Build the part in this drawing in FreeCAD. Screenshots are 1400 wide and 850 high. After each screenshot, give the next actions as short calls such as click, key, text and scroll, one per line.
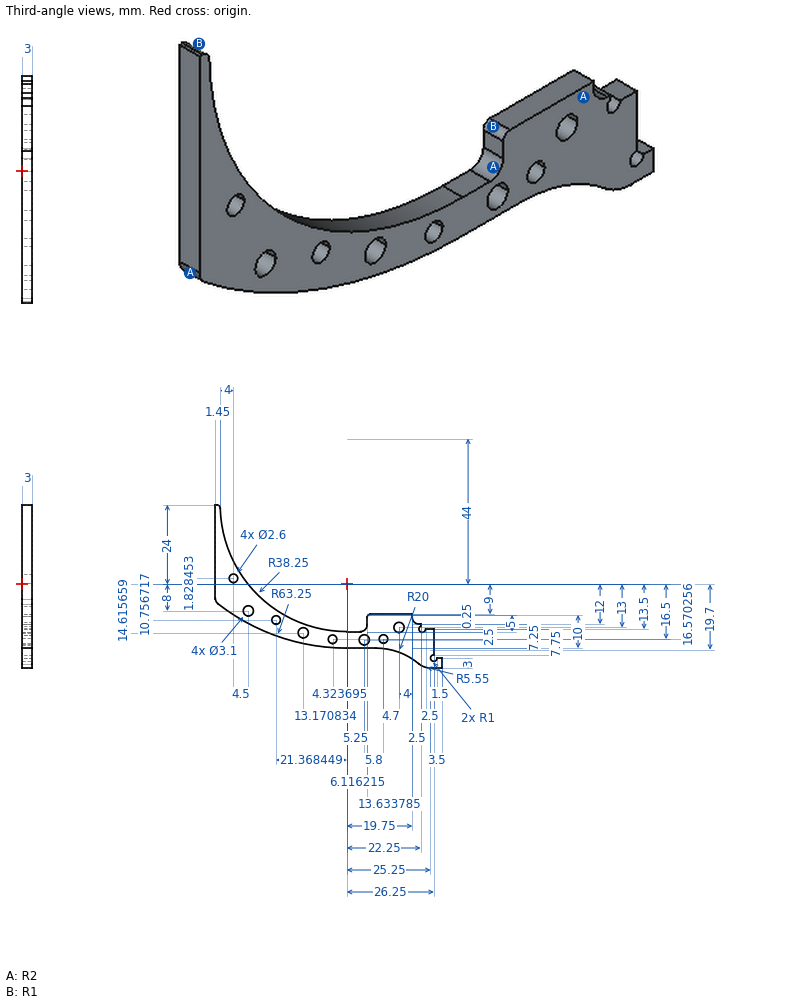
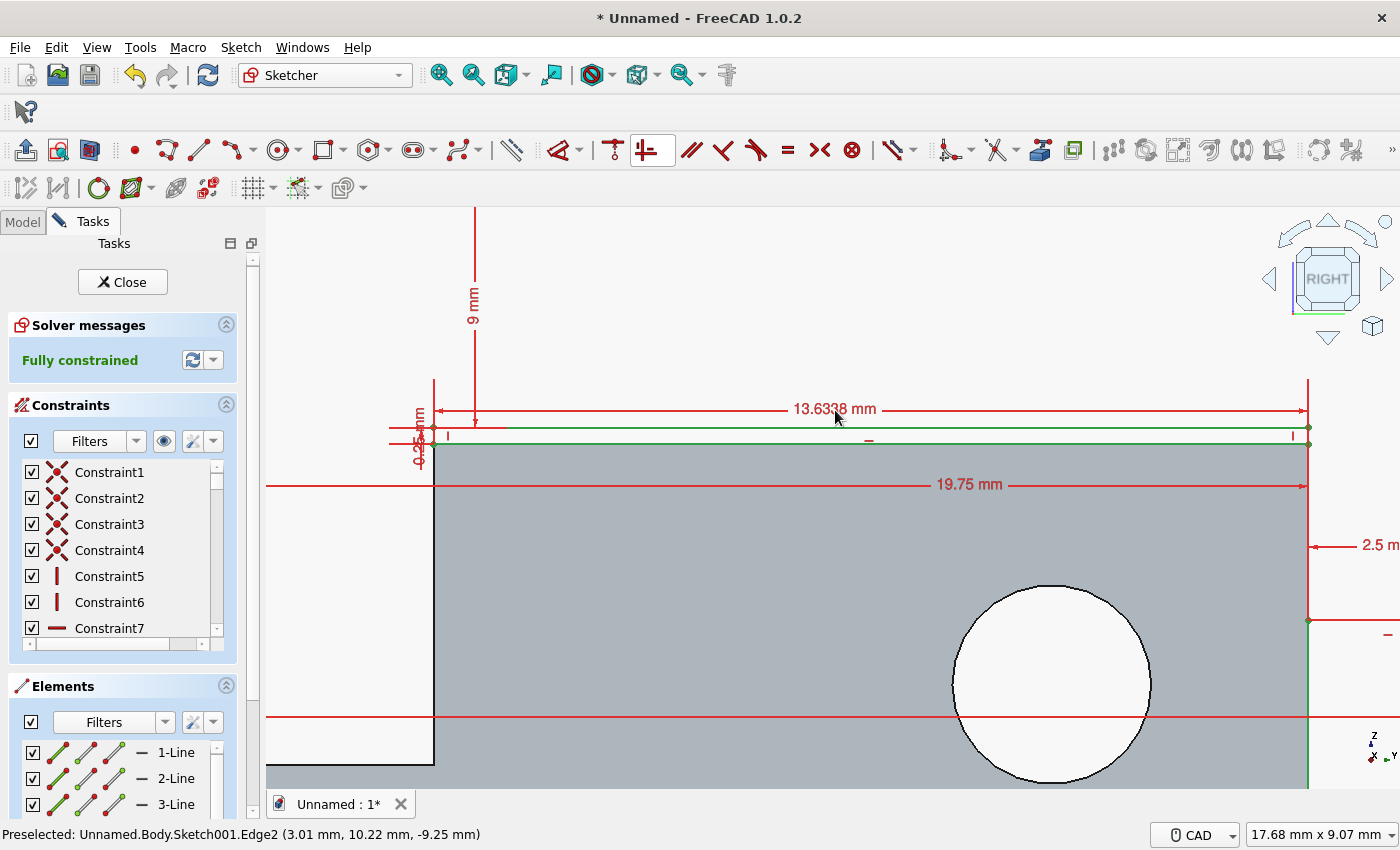
click(123, 282)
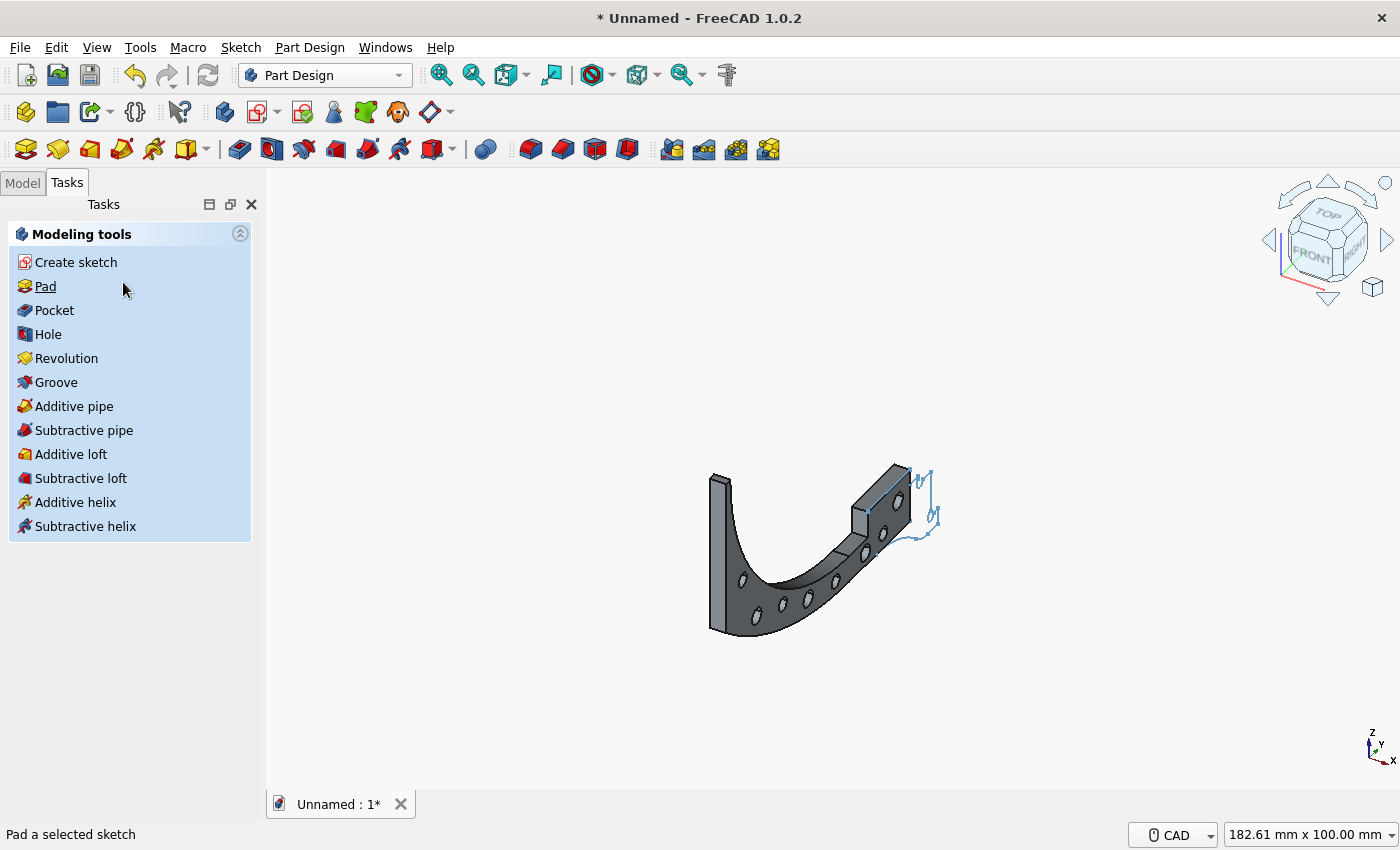
click(26, 150)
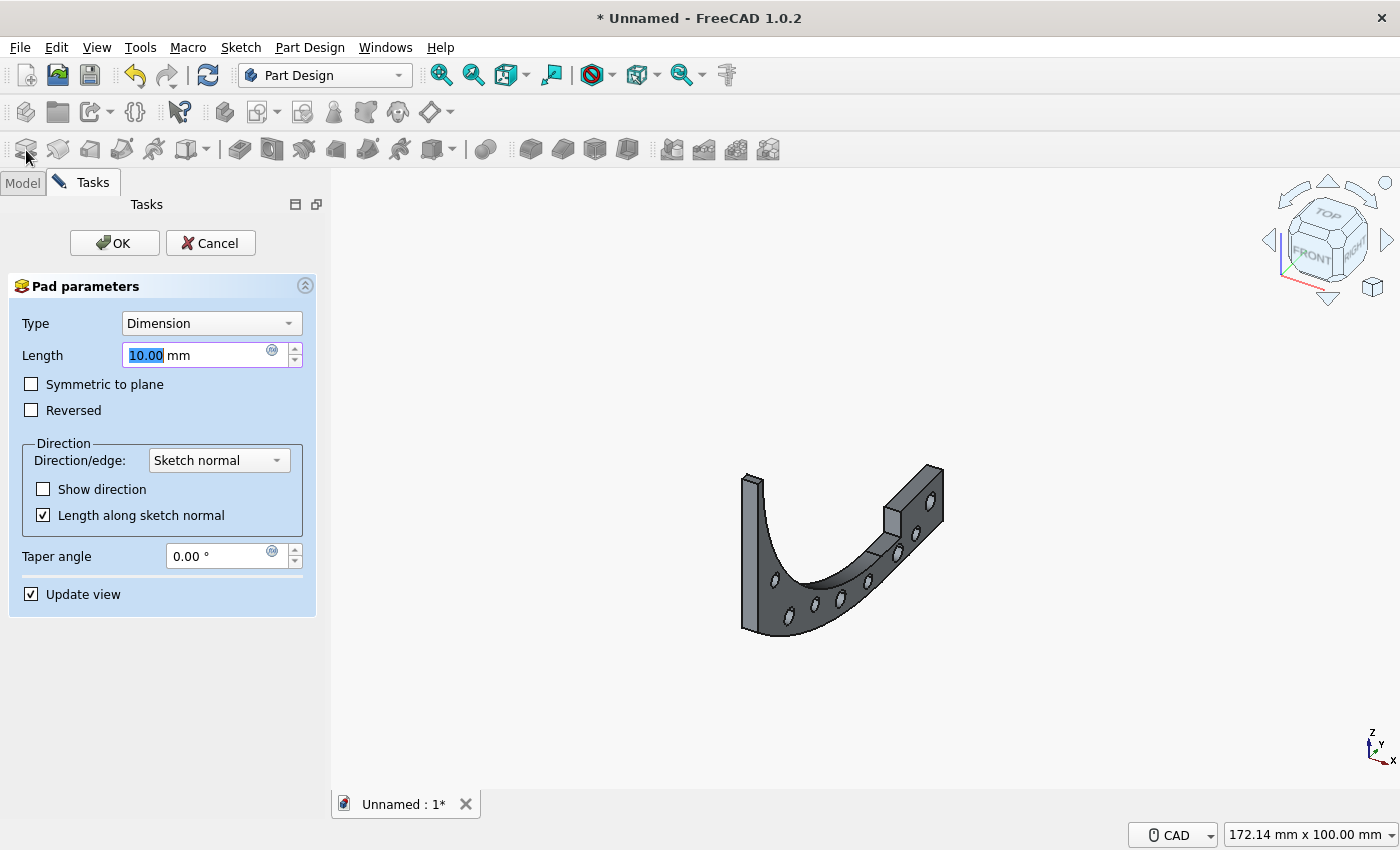
text(3)
key(Tab)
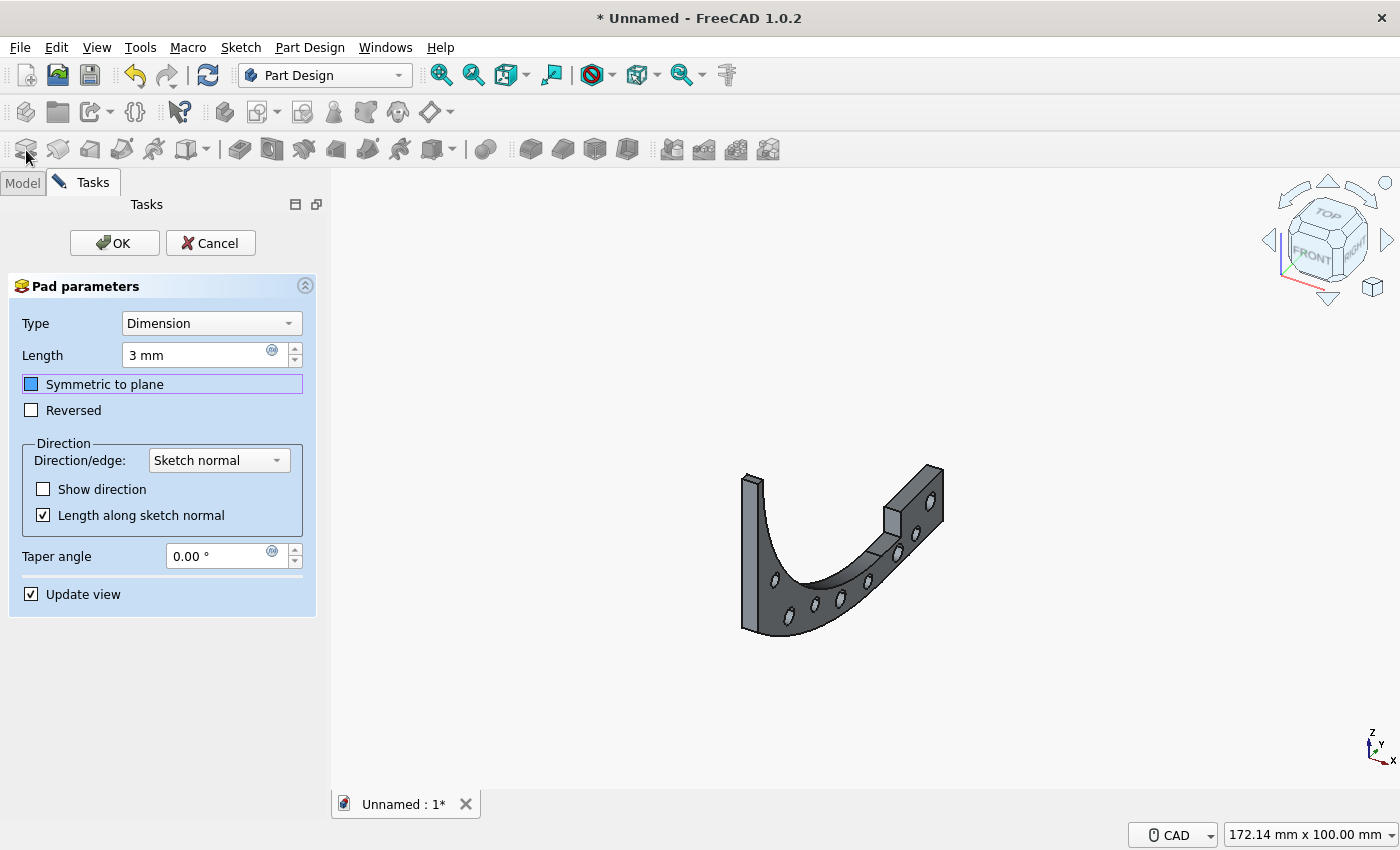
click(30, 410)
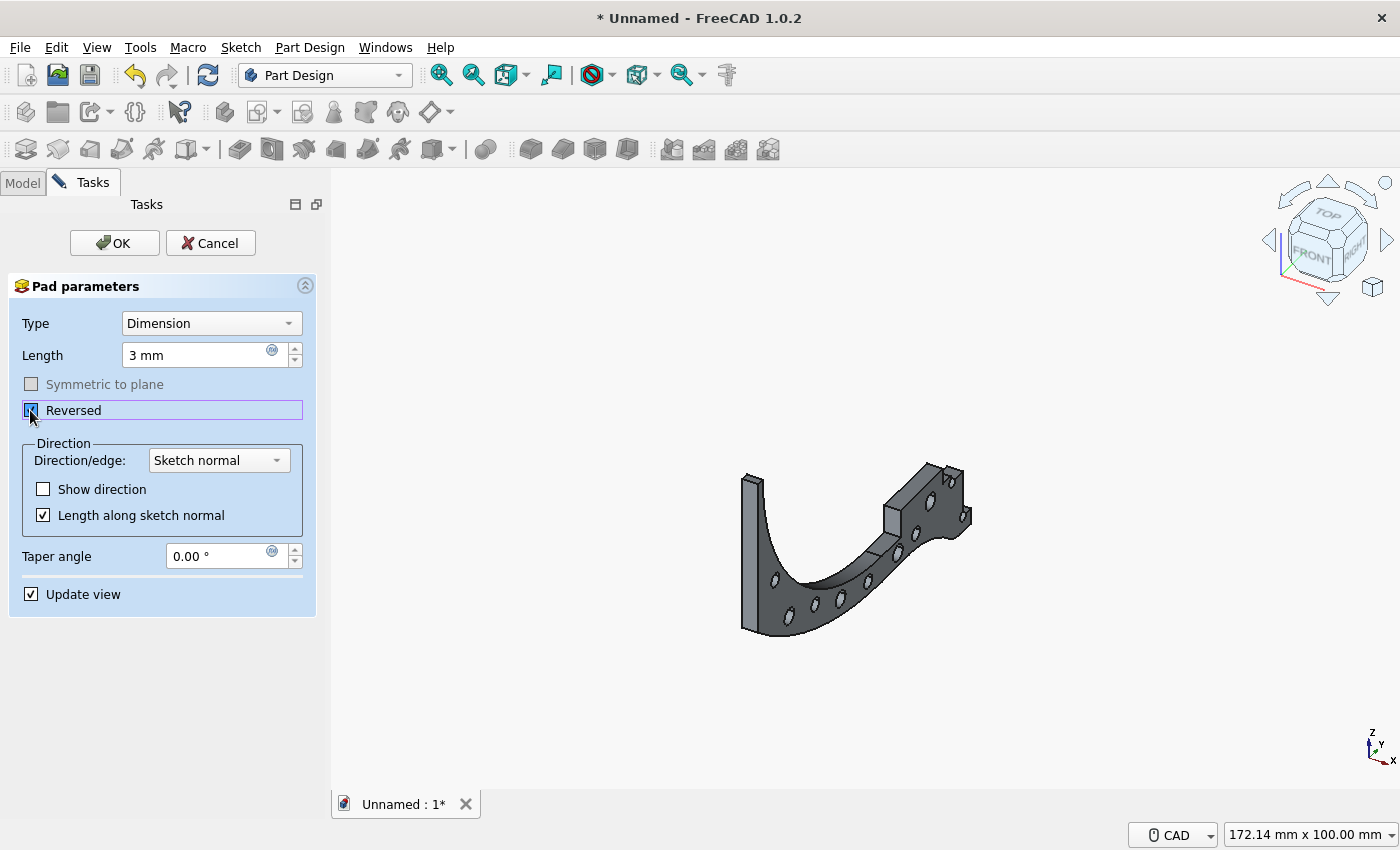
click(115, 243)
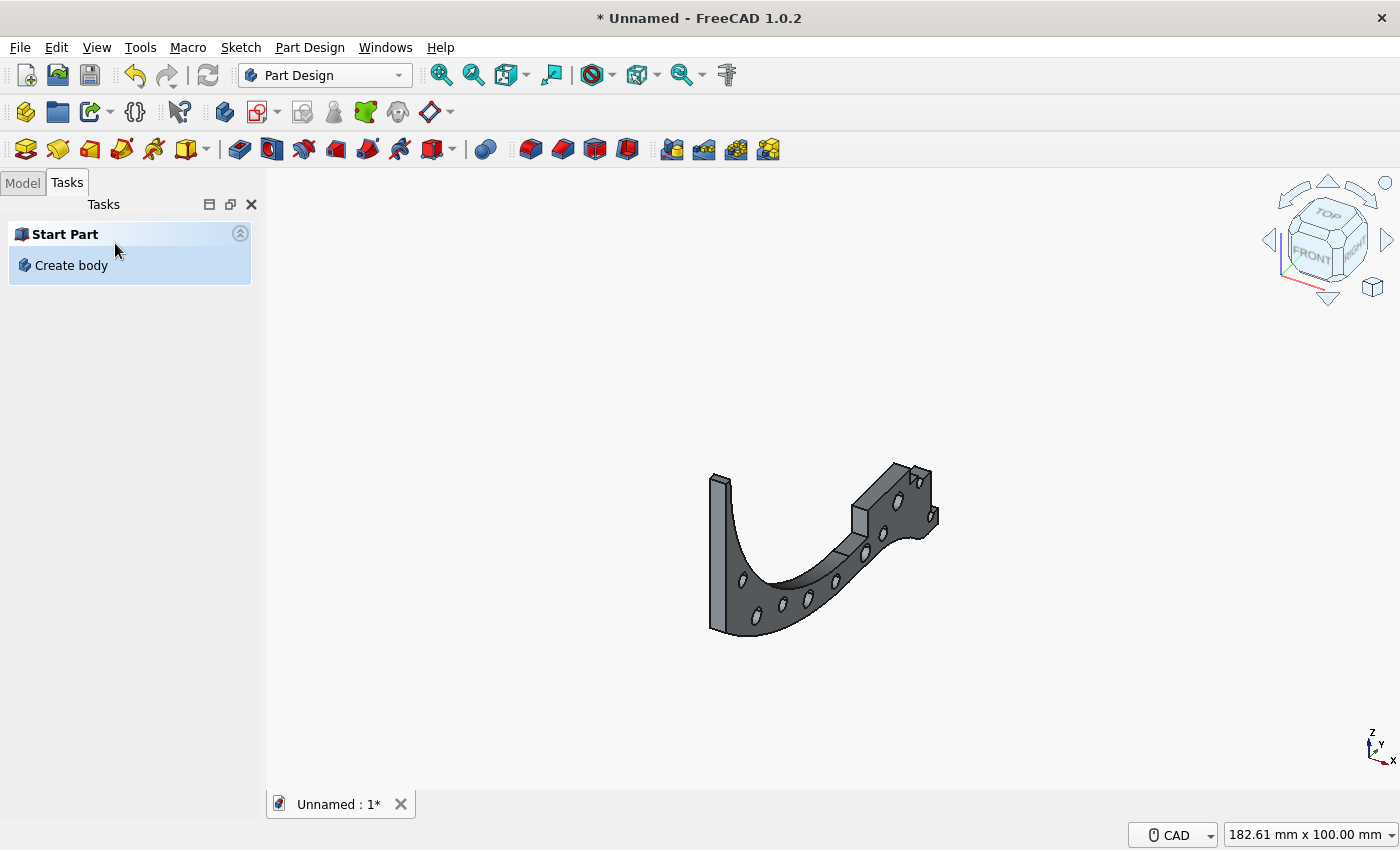
scroll(718, 629, up, 4)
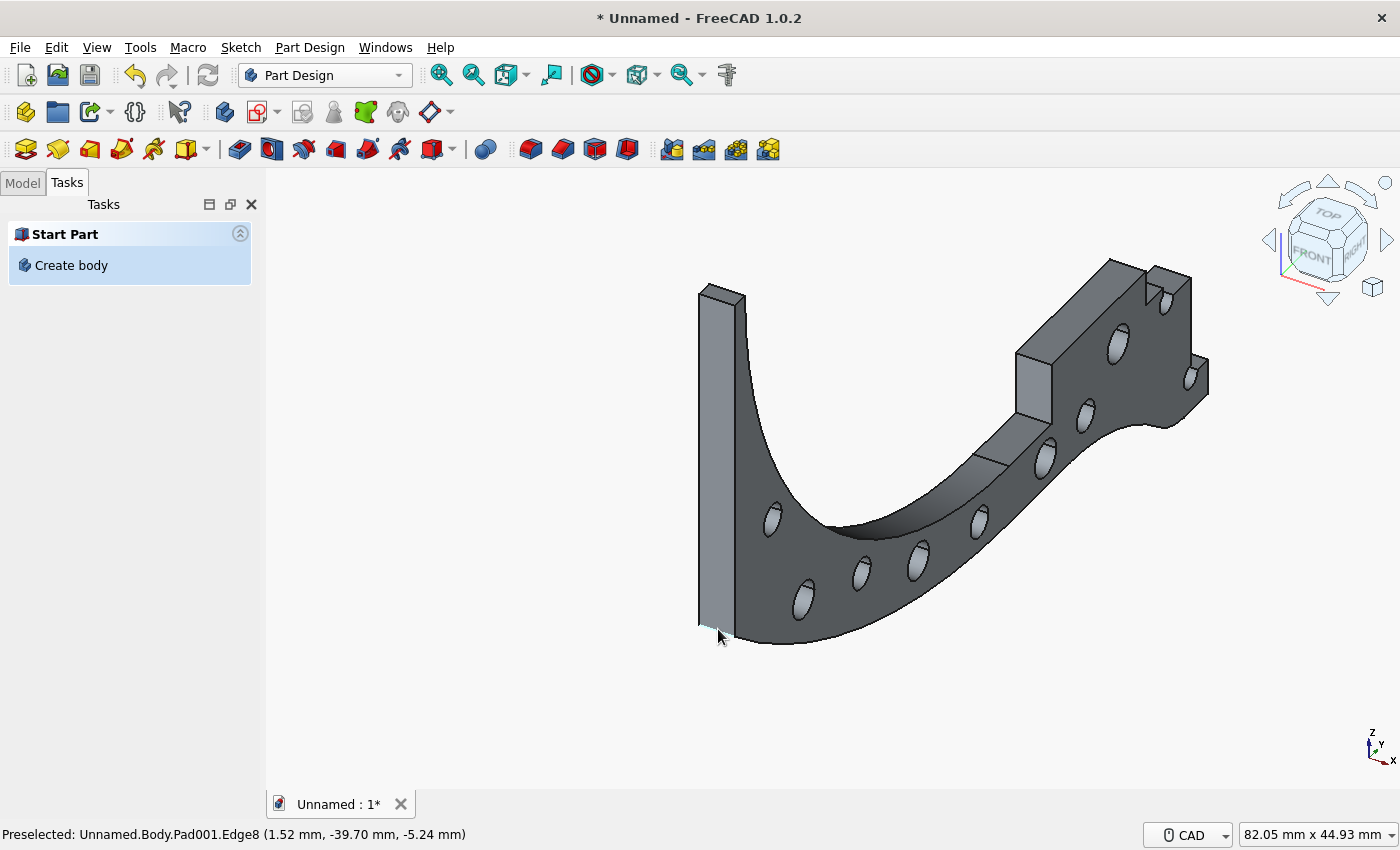
key(v)
key(f)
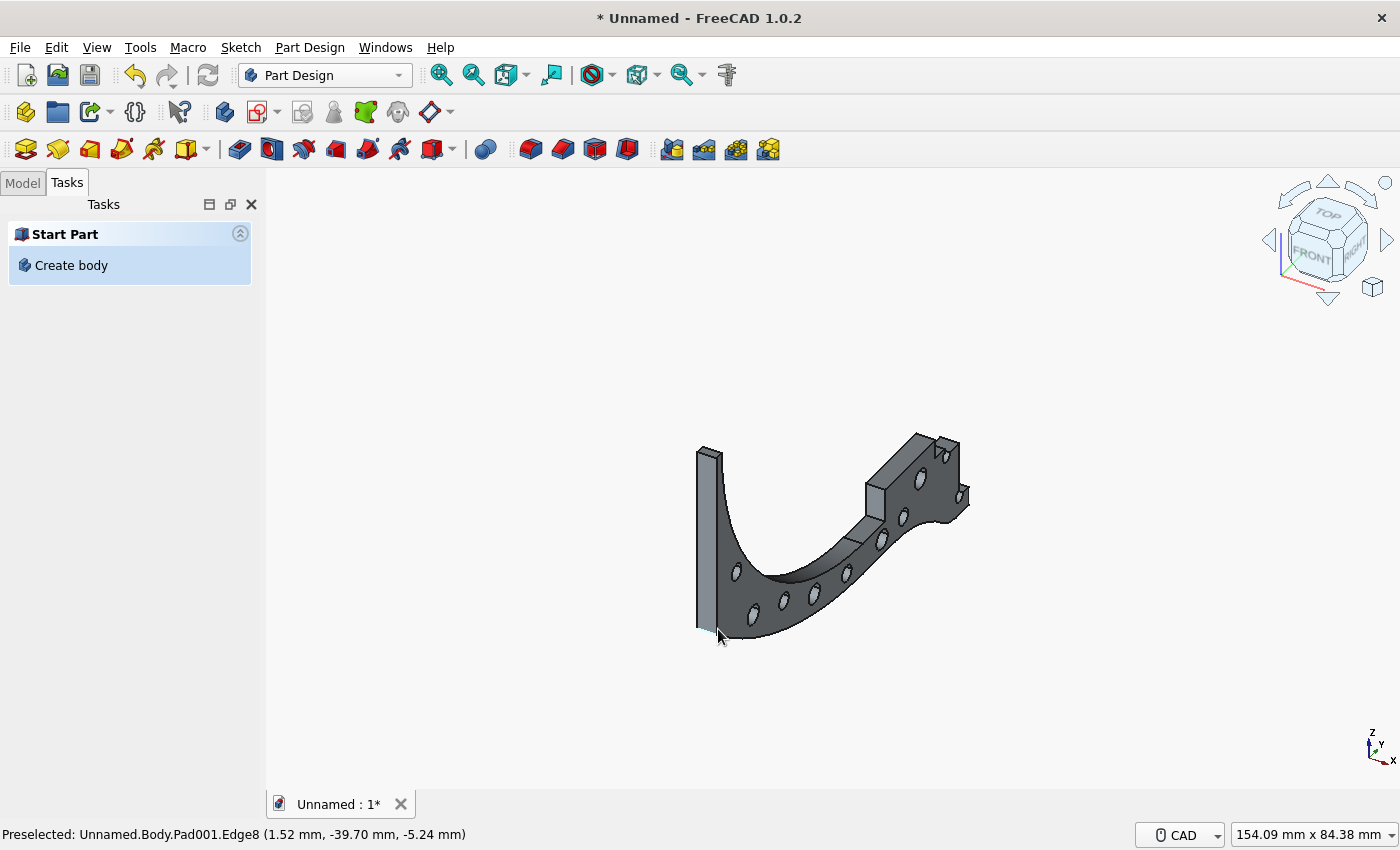
key(0)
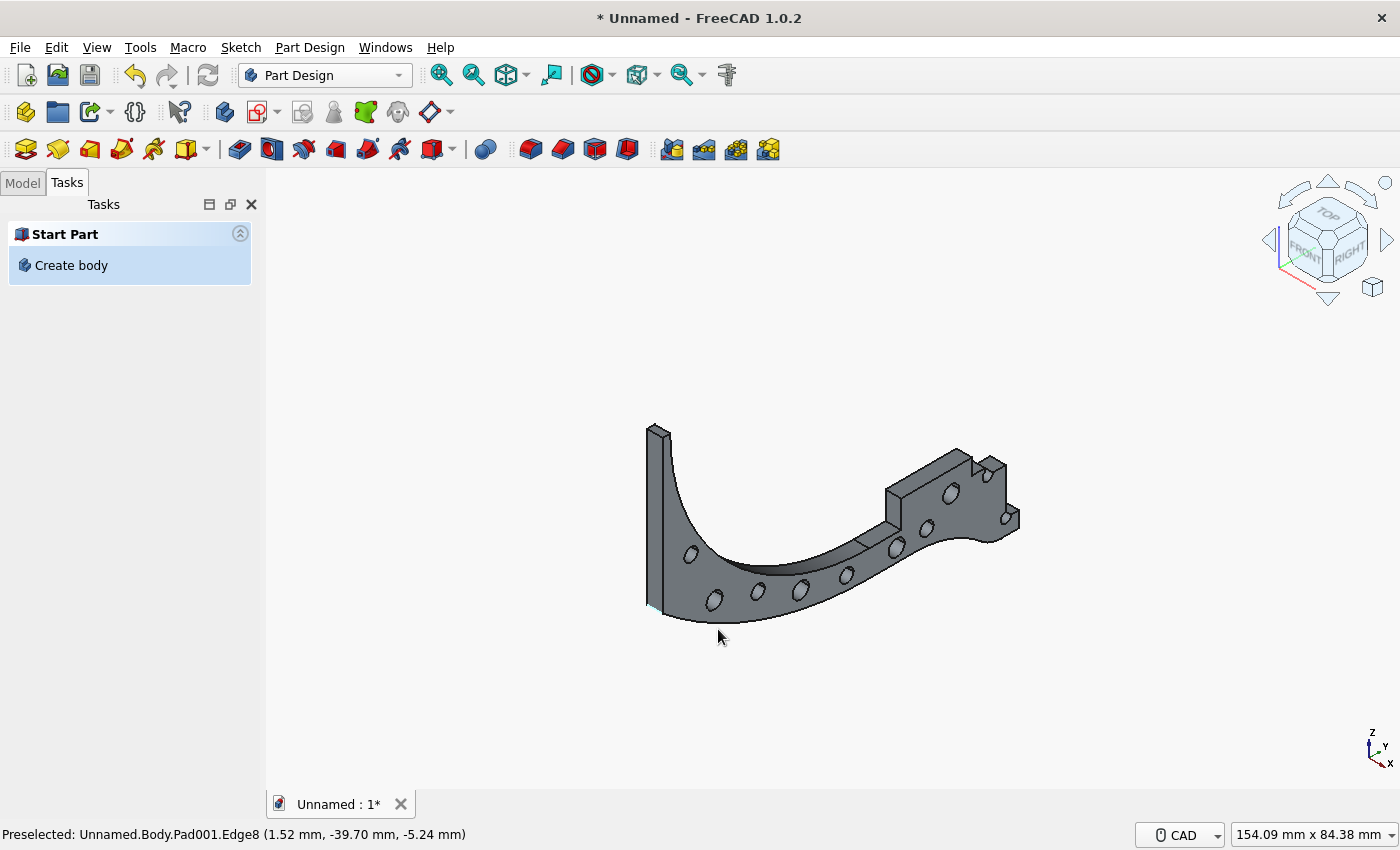
key(2)